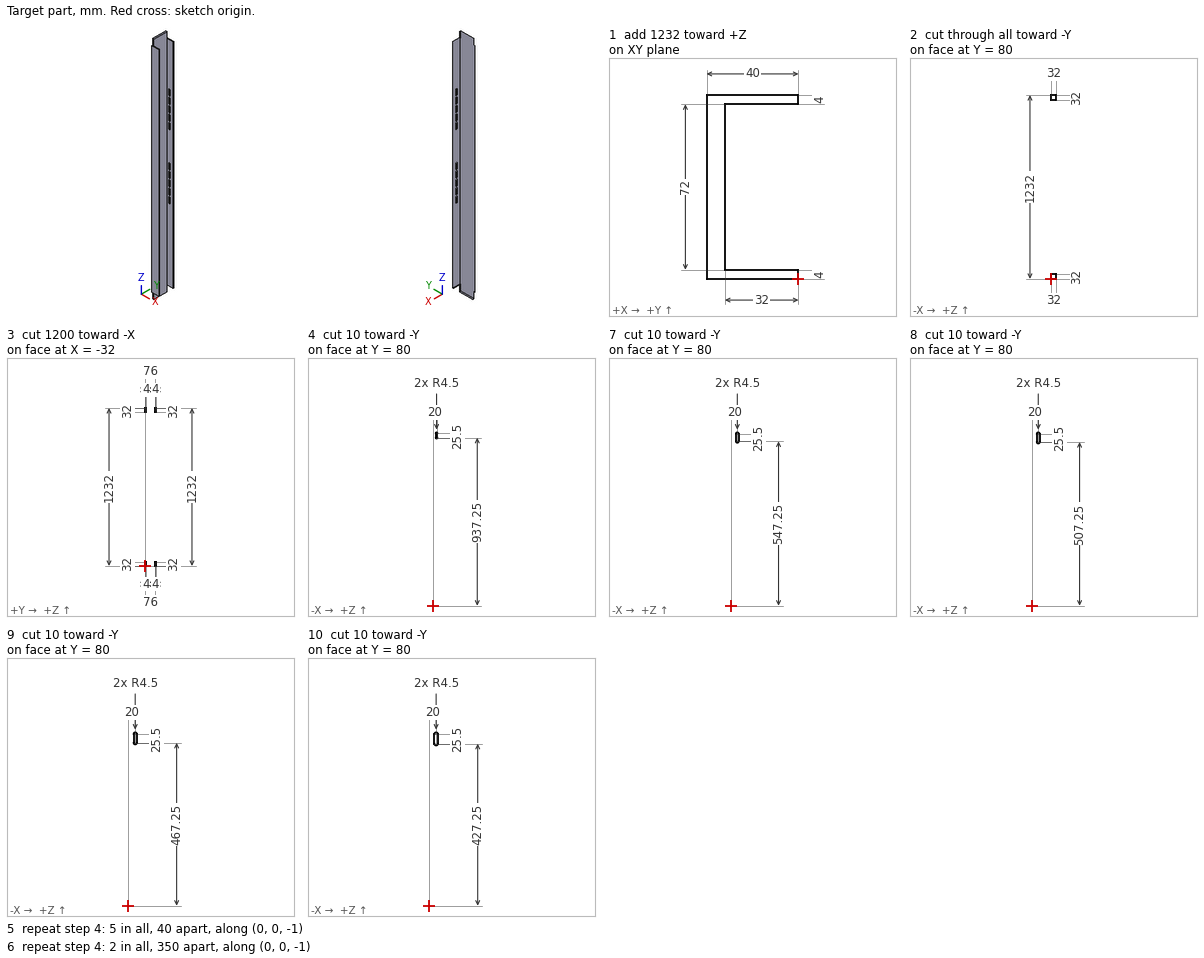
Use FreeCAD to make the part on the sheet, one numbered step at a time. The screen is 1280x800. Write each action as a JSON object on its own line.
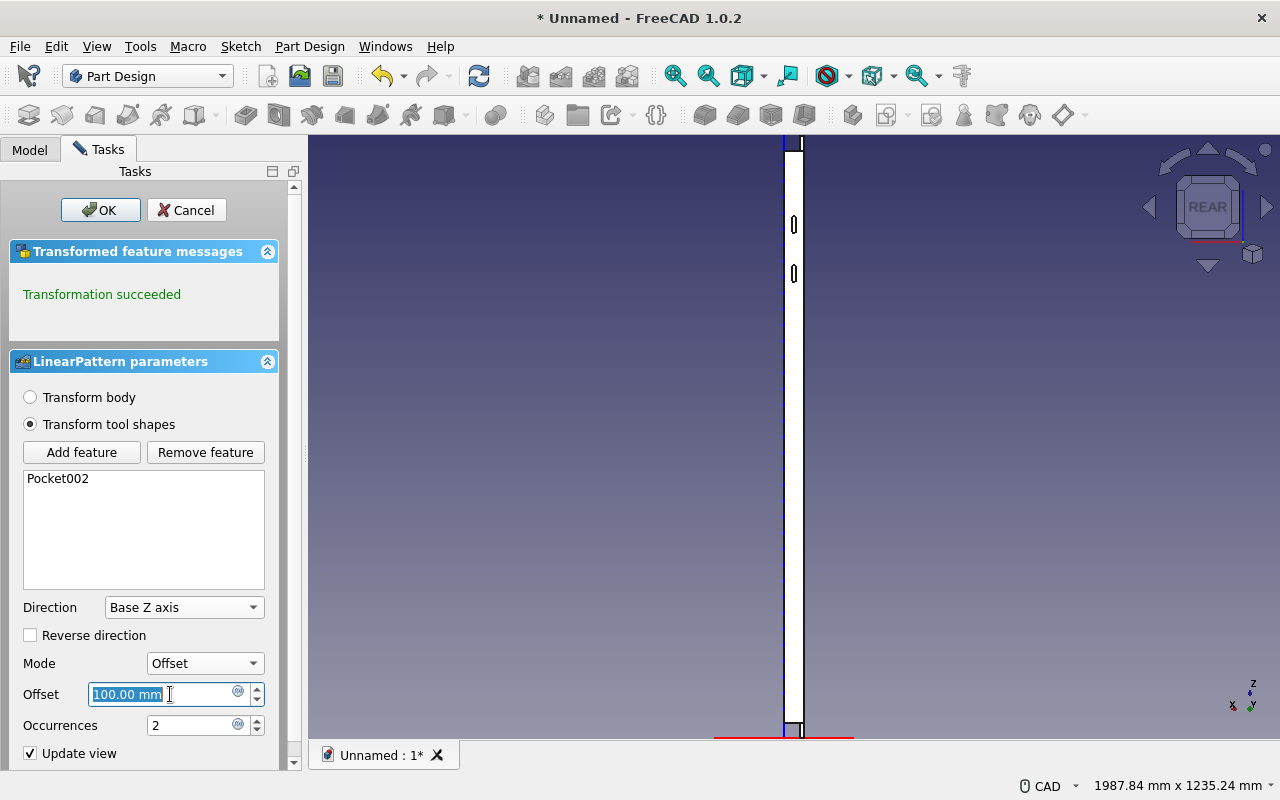
{"action": "type", "text": "40"}
{"action": "key", "text": "Tab"}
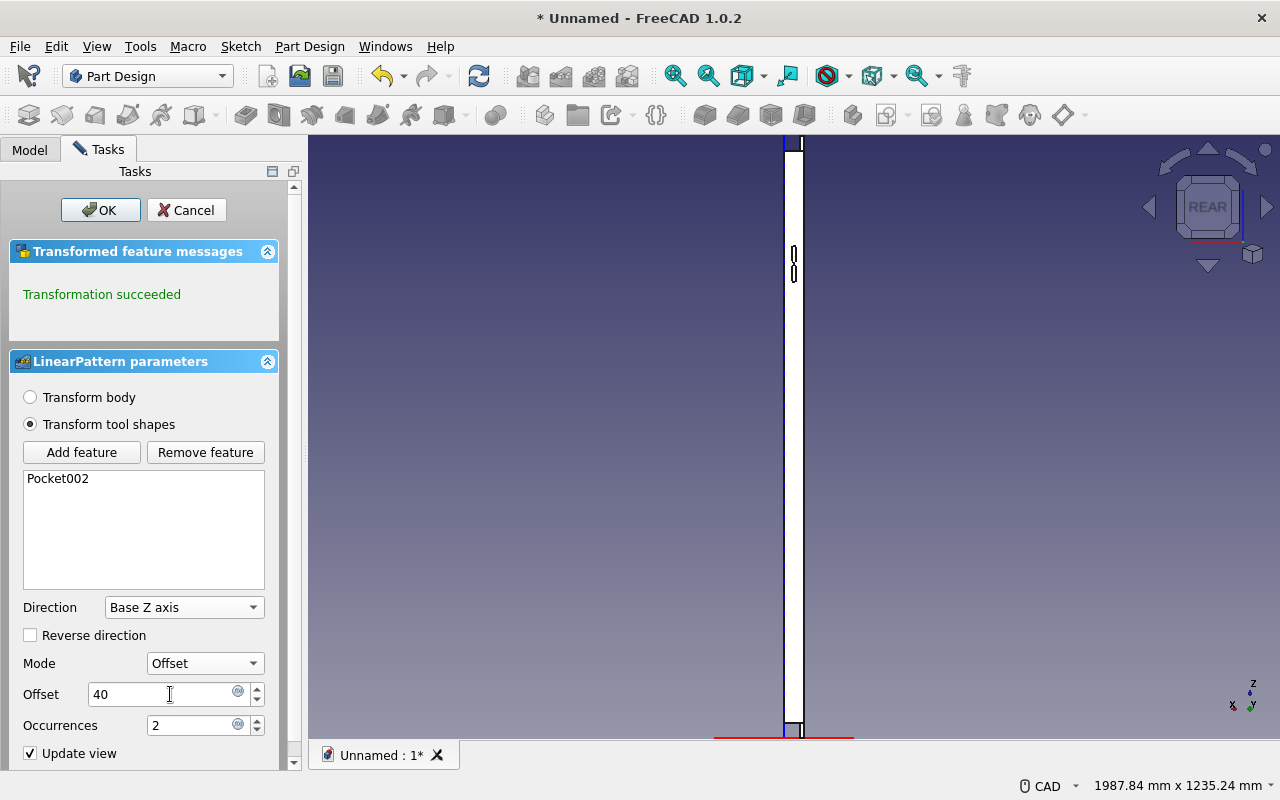
{"action": "triple_click", "coordinate": [199, 726]}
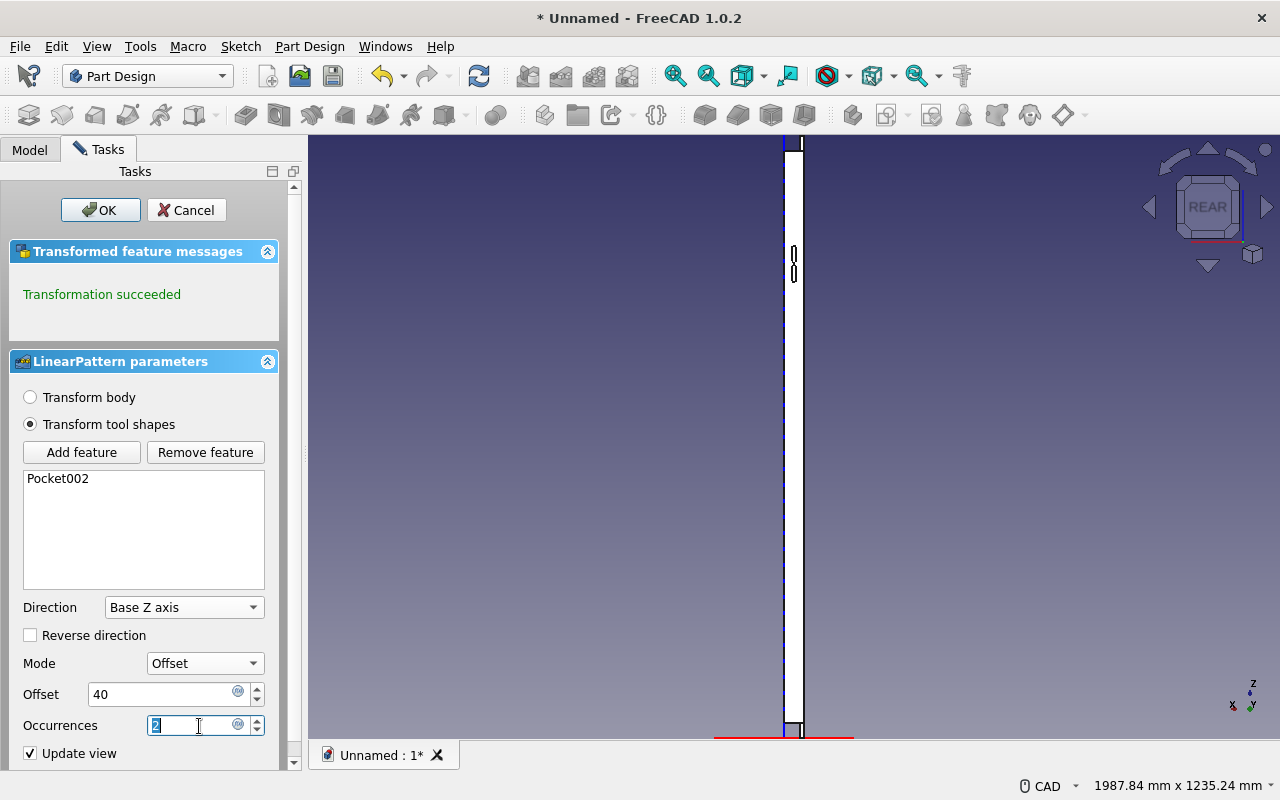
{"action": "type", "text": "5"}
{"action": "key", "text": "Tab"}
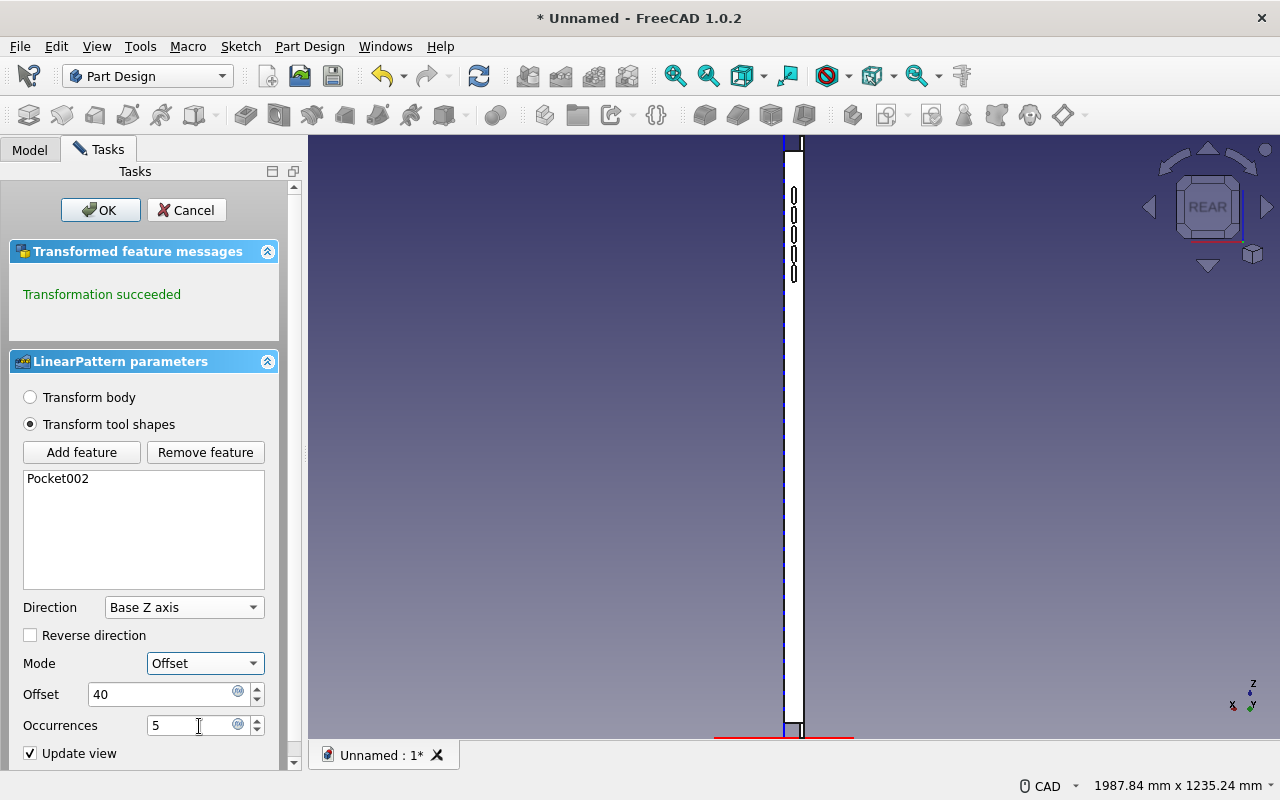
{"action": "left_click", "coordinate": [31, 635]}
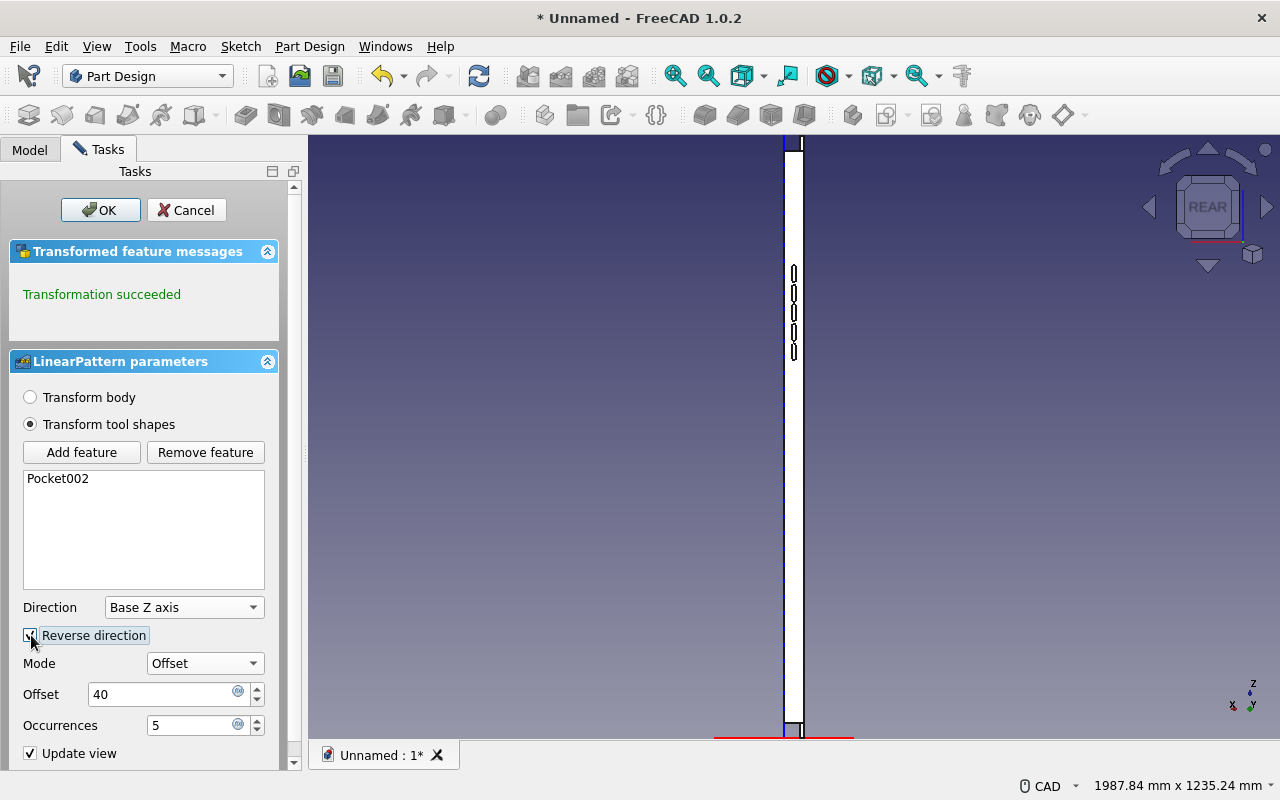
{"action": "left_click", "coordinate": [101, 210]}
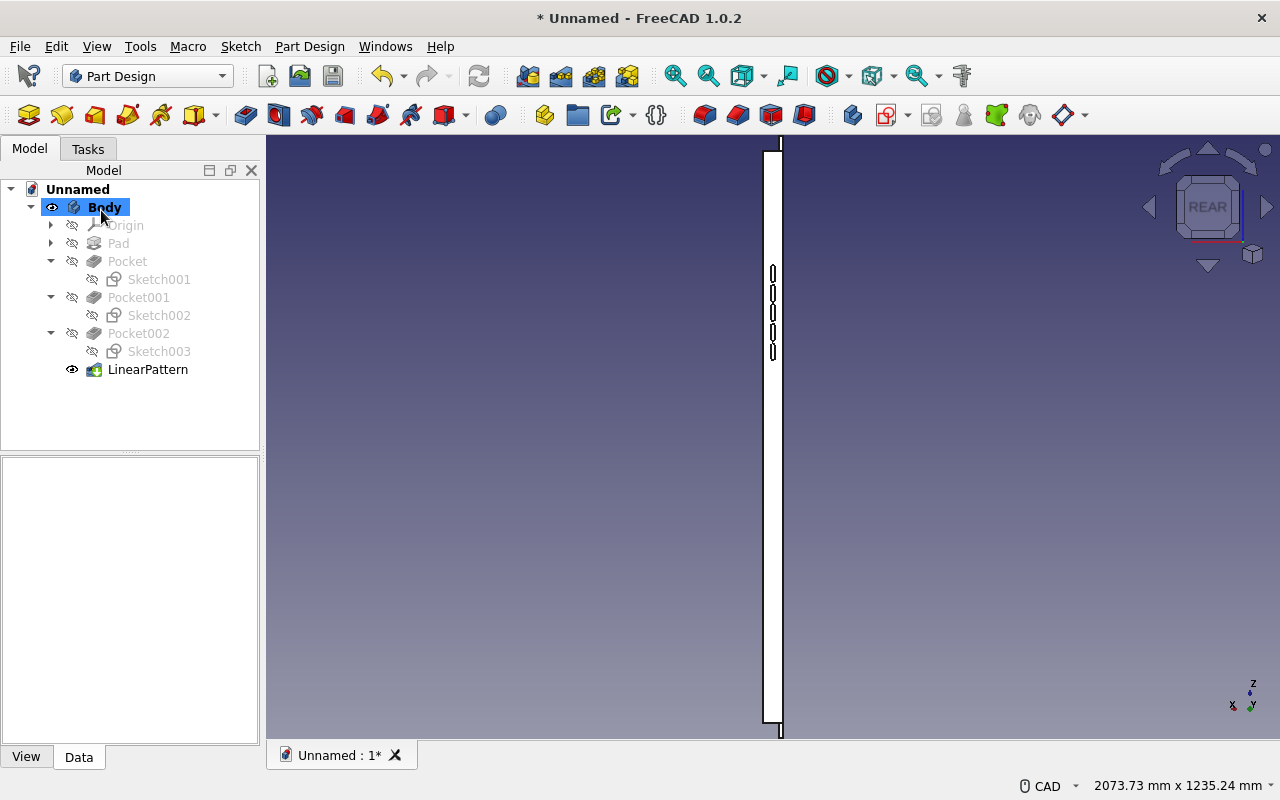
{"action": "left_click", "coordinate": [117, 333]}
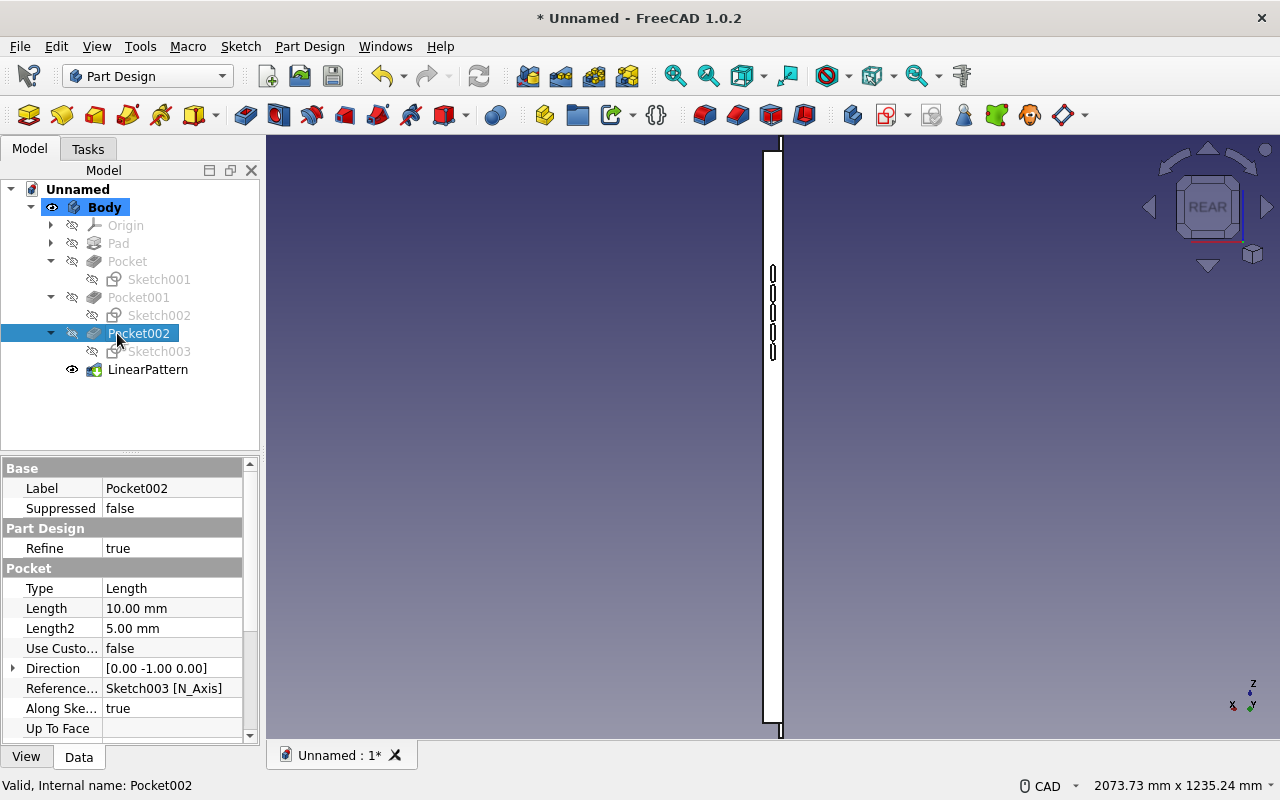
{"action": "left_click", "coordinate": [561, 76]}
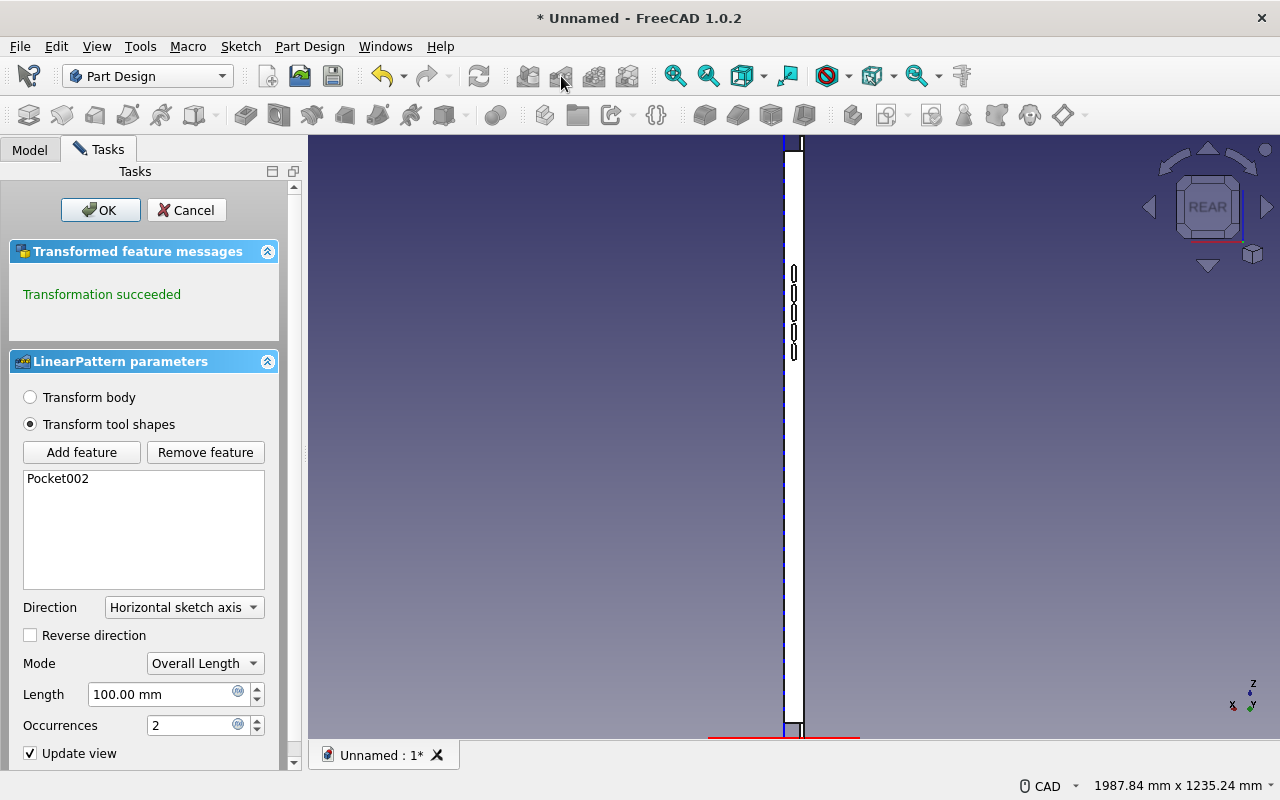
{"action": "left_click", "coordinate": [185, 608]}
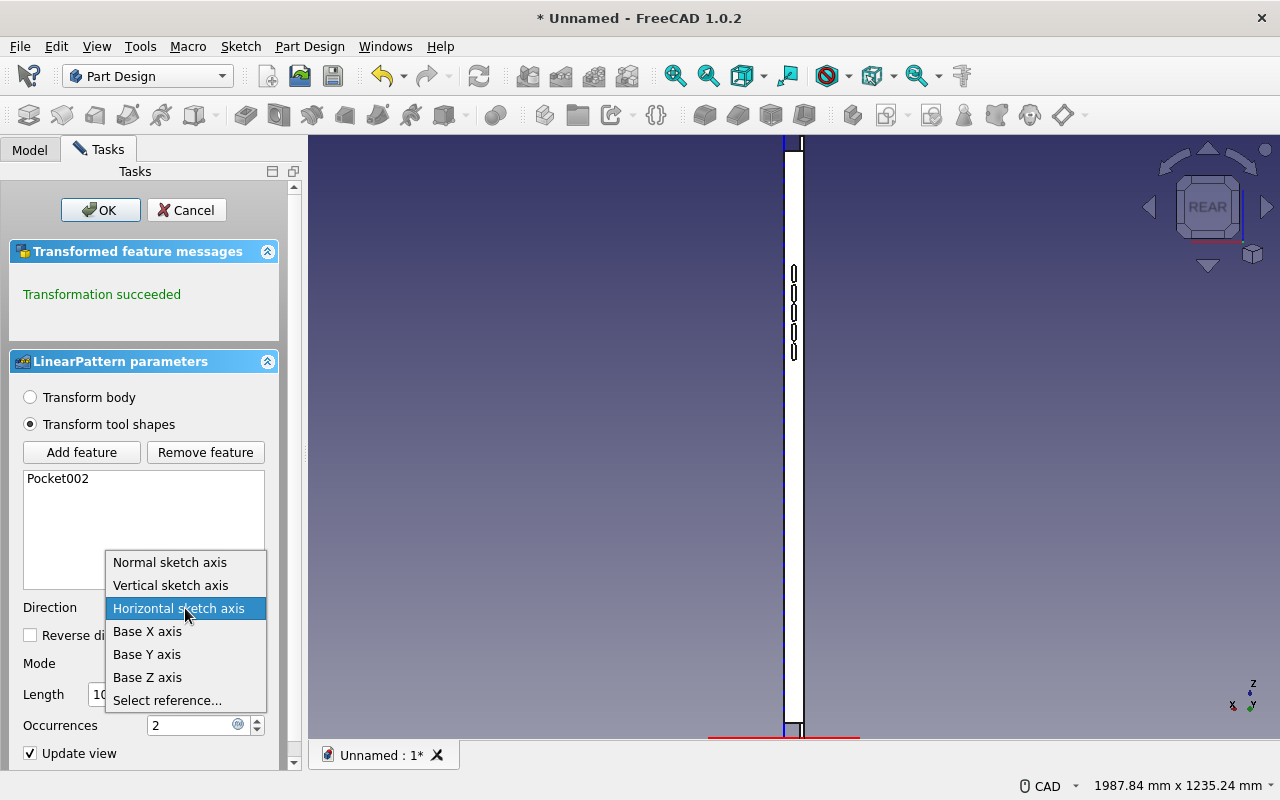
{"action": "left_click", "coordinate": [184, 678]}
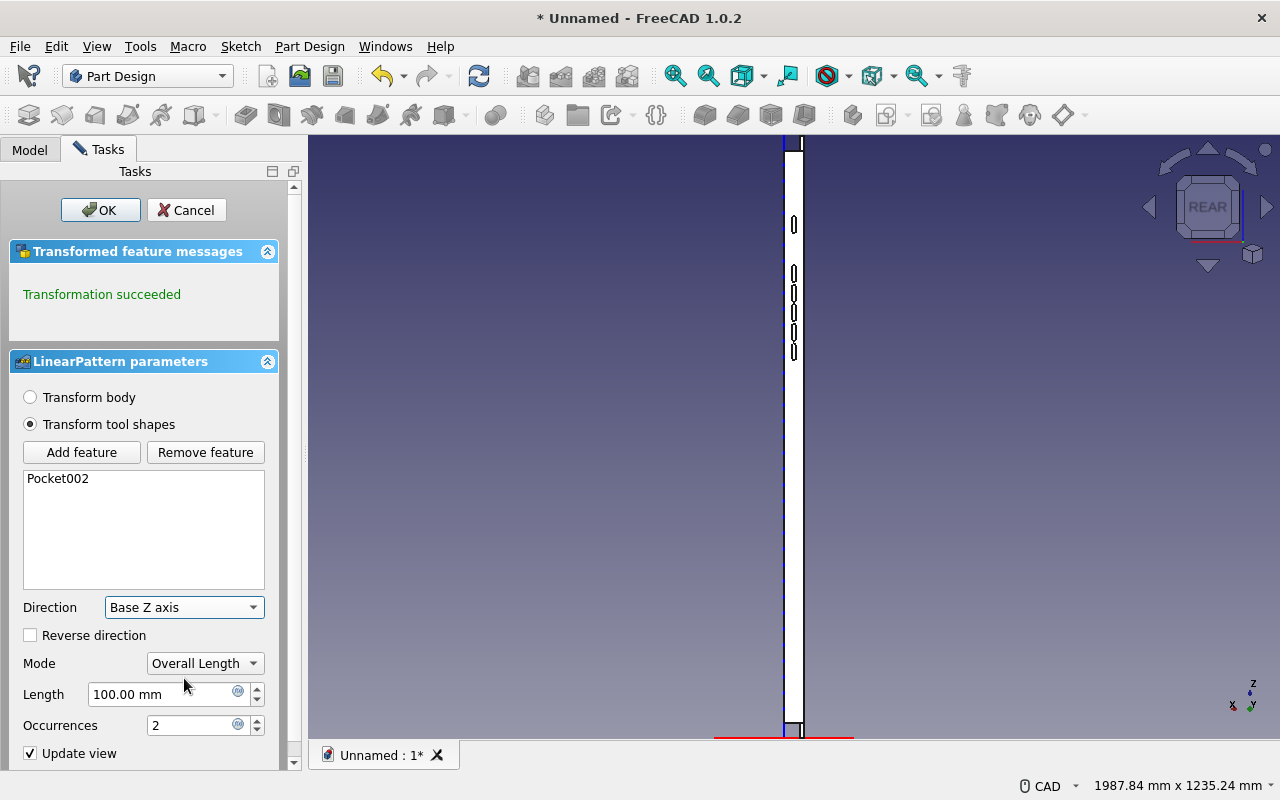
{"action": "left_click", "coordinate": [206, 664]}